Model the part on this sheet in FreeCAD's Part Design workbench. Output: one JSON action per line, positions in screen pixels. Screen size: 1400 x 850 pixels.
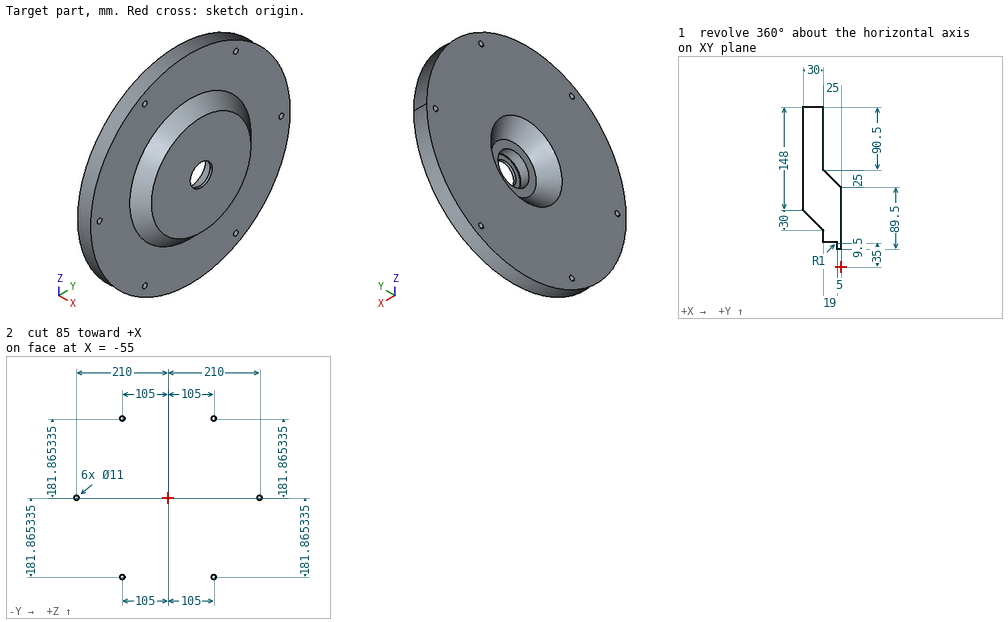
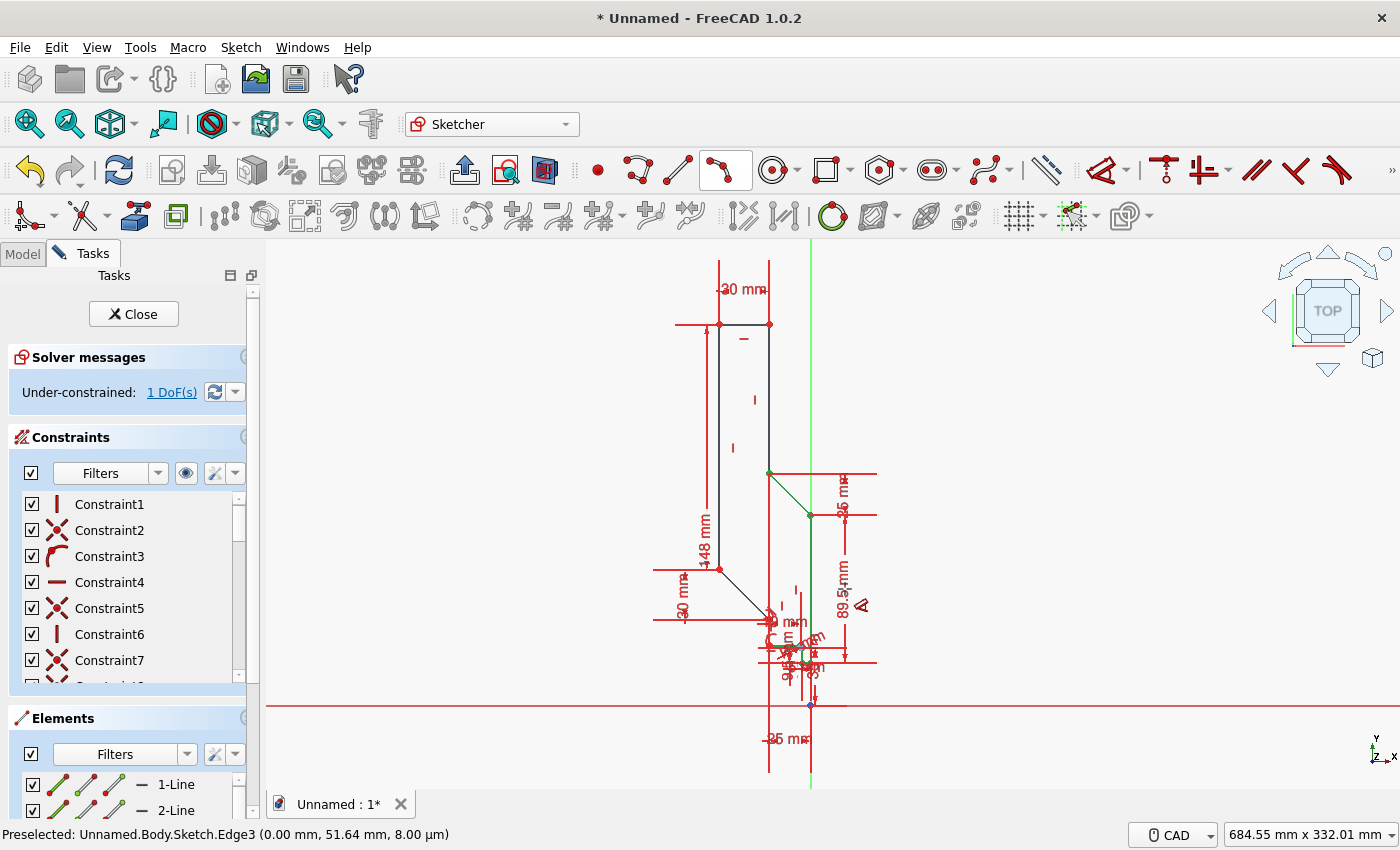
{"action": "left_click", "coordinate": [769, 429]}
{"action": "left_click", "coordinate": [735, 399]}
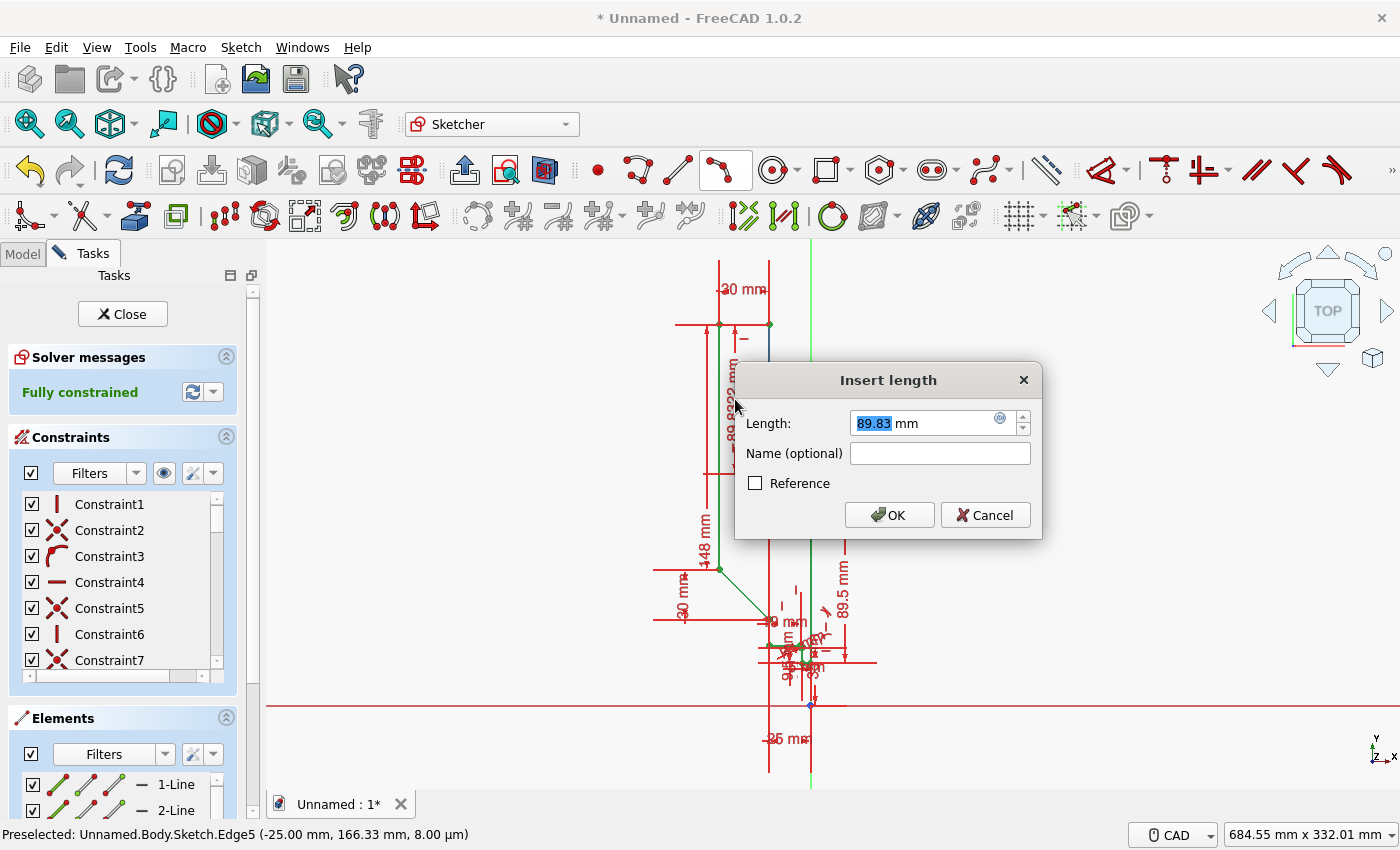
{"action": "type", "text": "90.5"}
{"action": "key", "text": "Return"}
{"action": "key", "text": "Escape"}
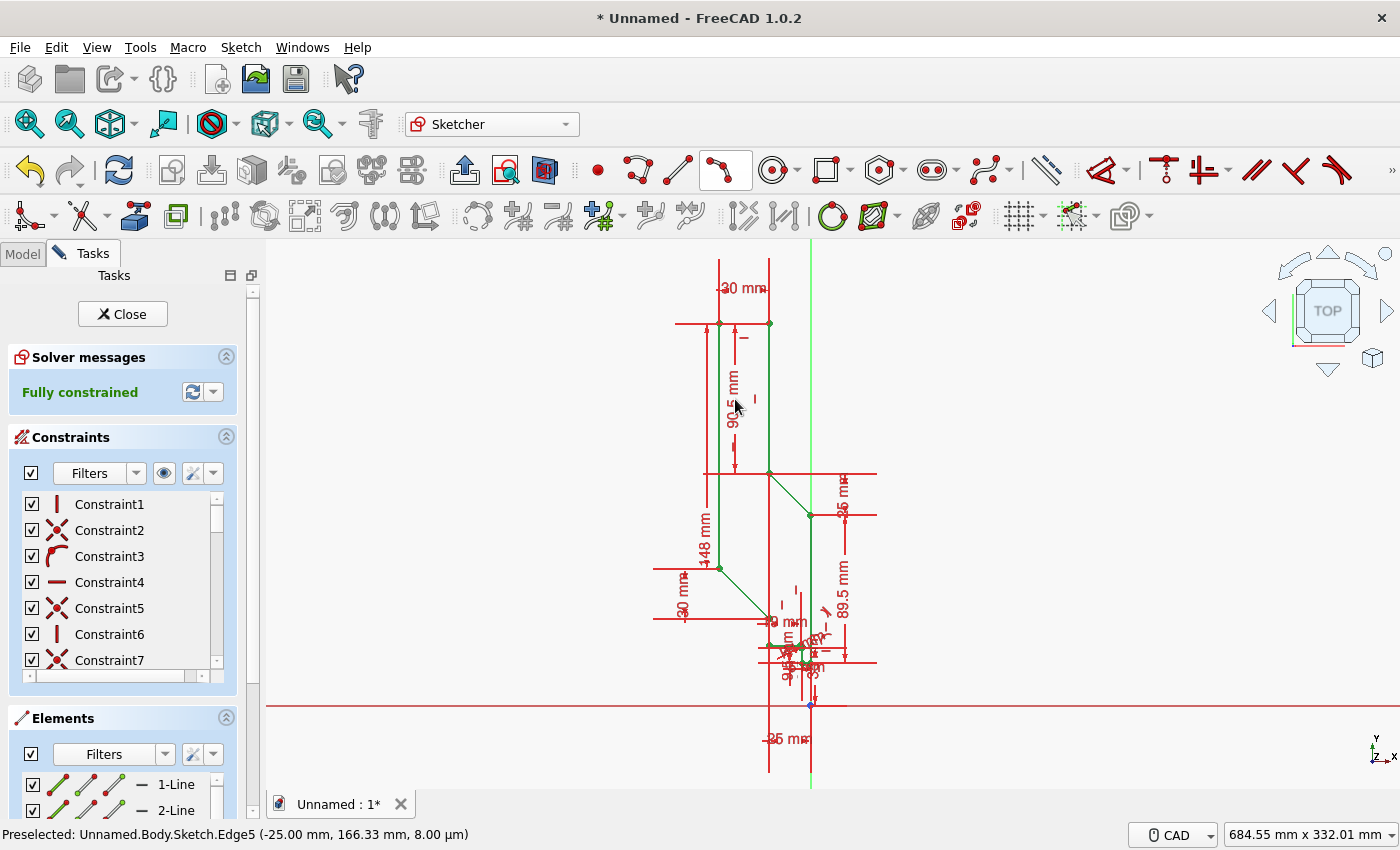
{"action": "left_click", "coordinate": [123, 314]}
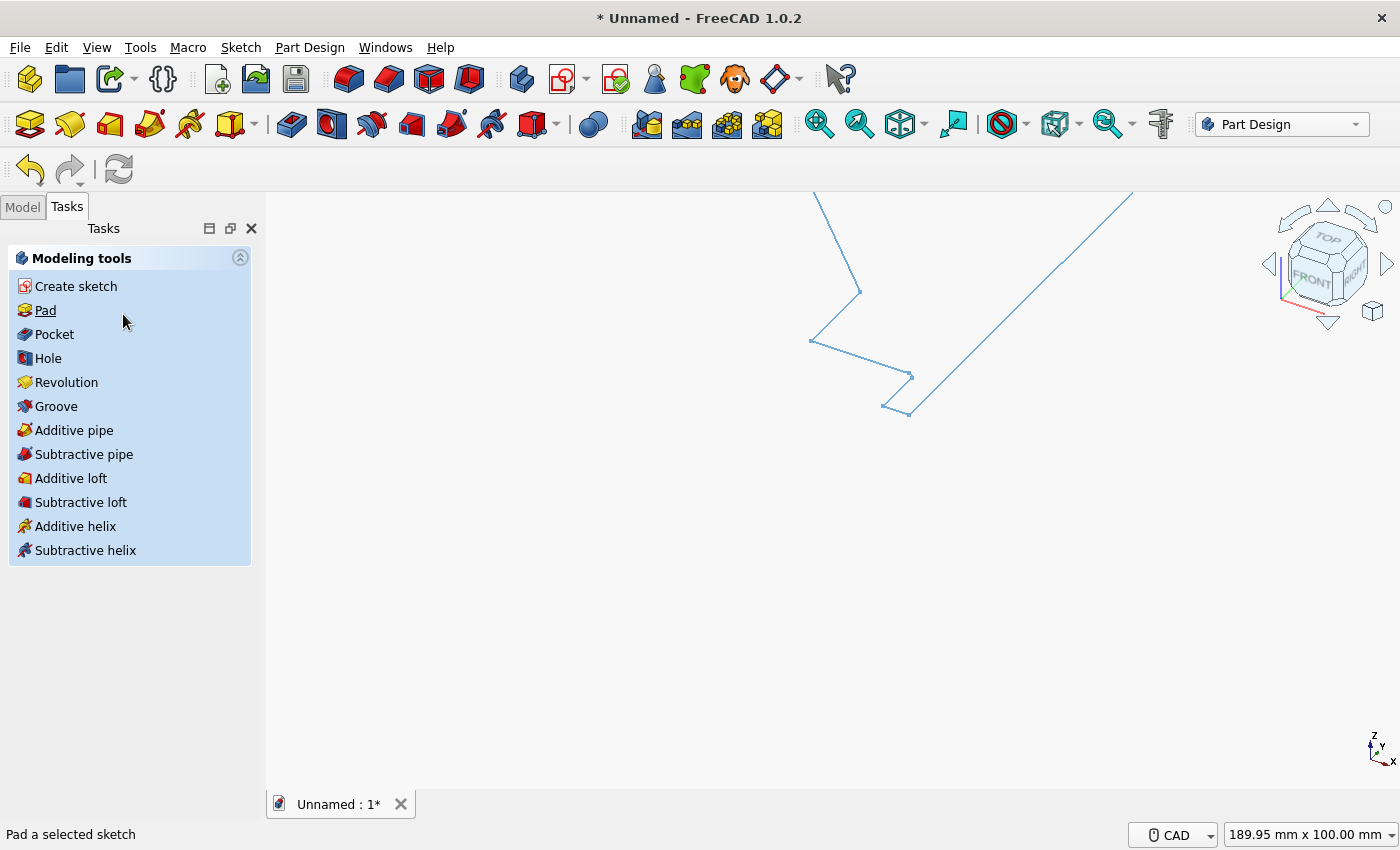
{"action": "left_click", "coordinate": [70, 124]}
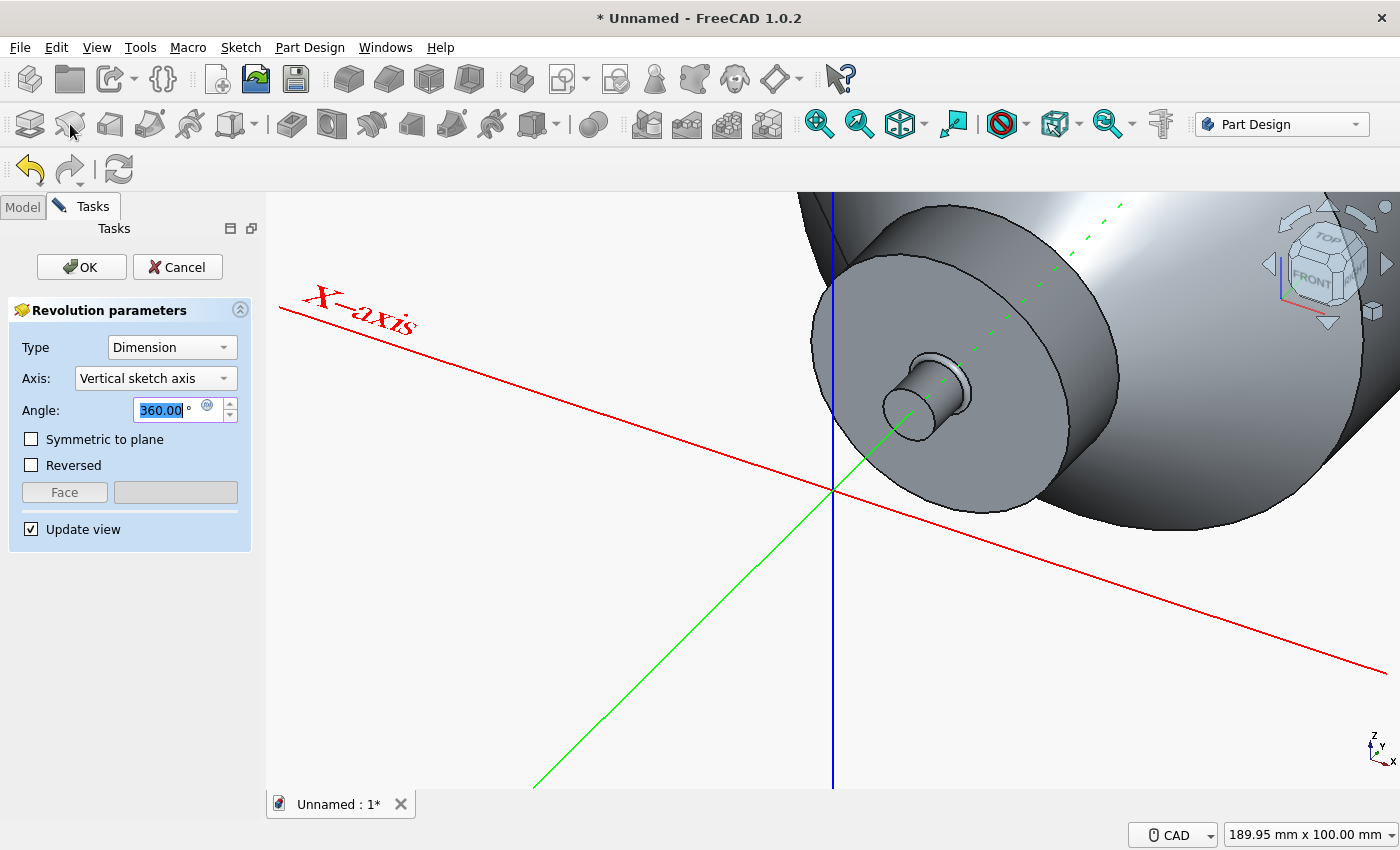
{"action": "left_click", "coordinate": [156, 378]}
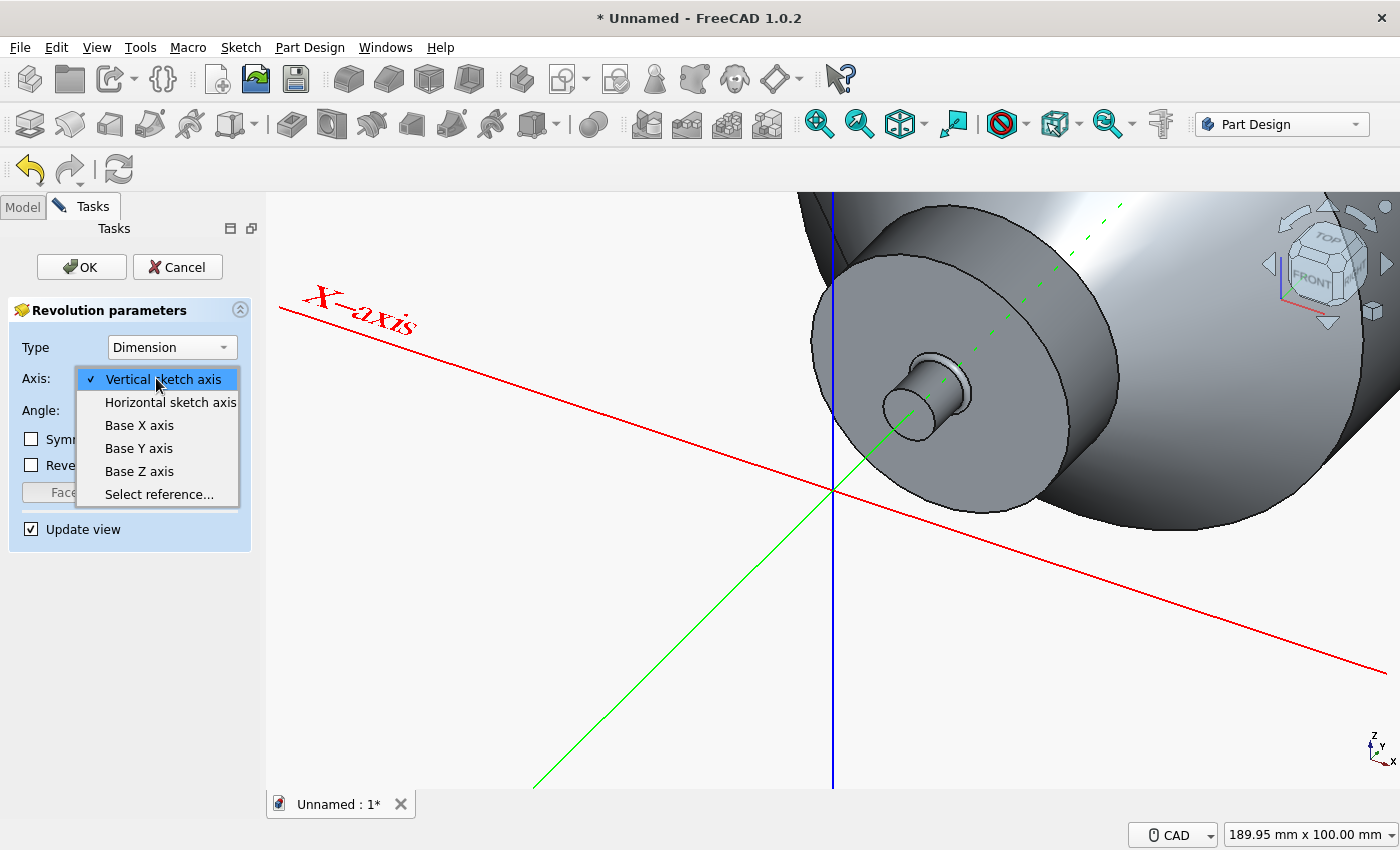
{"action": "left_click", "coordinate": [156, 402]}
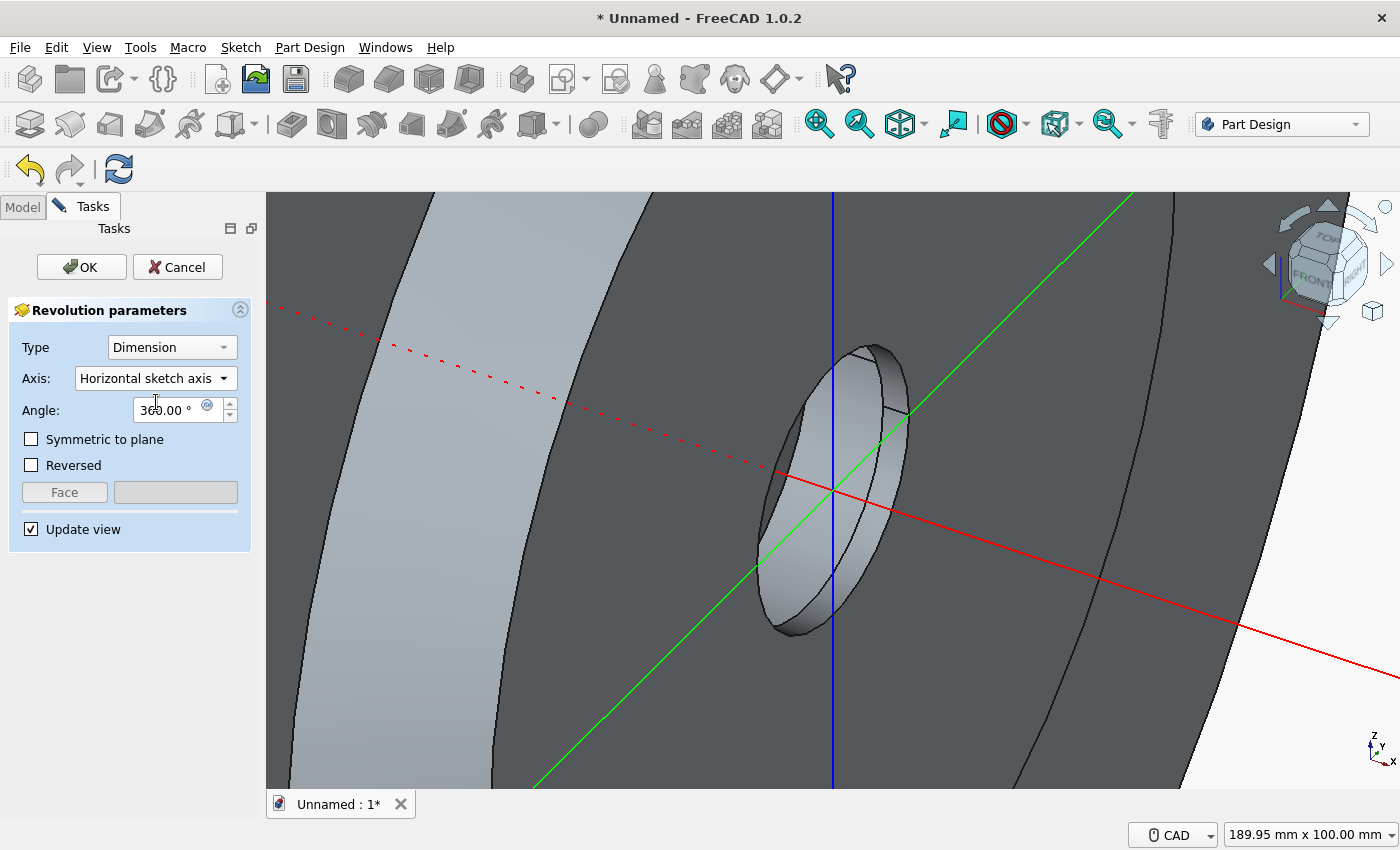
{"action": "left_click", "coordinate": [82, 267]}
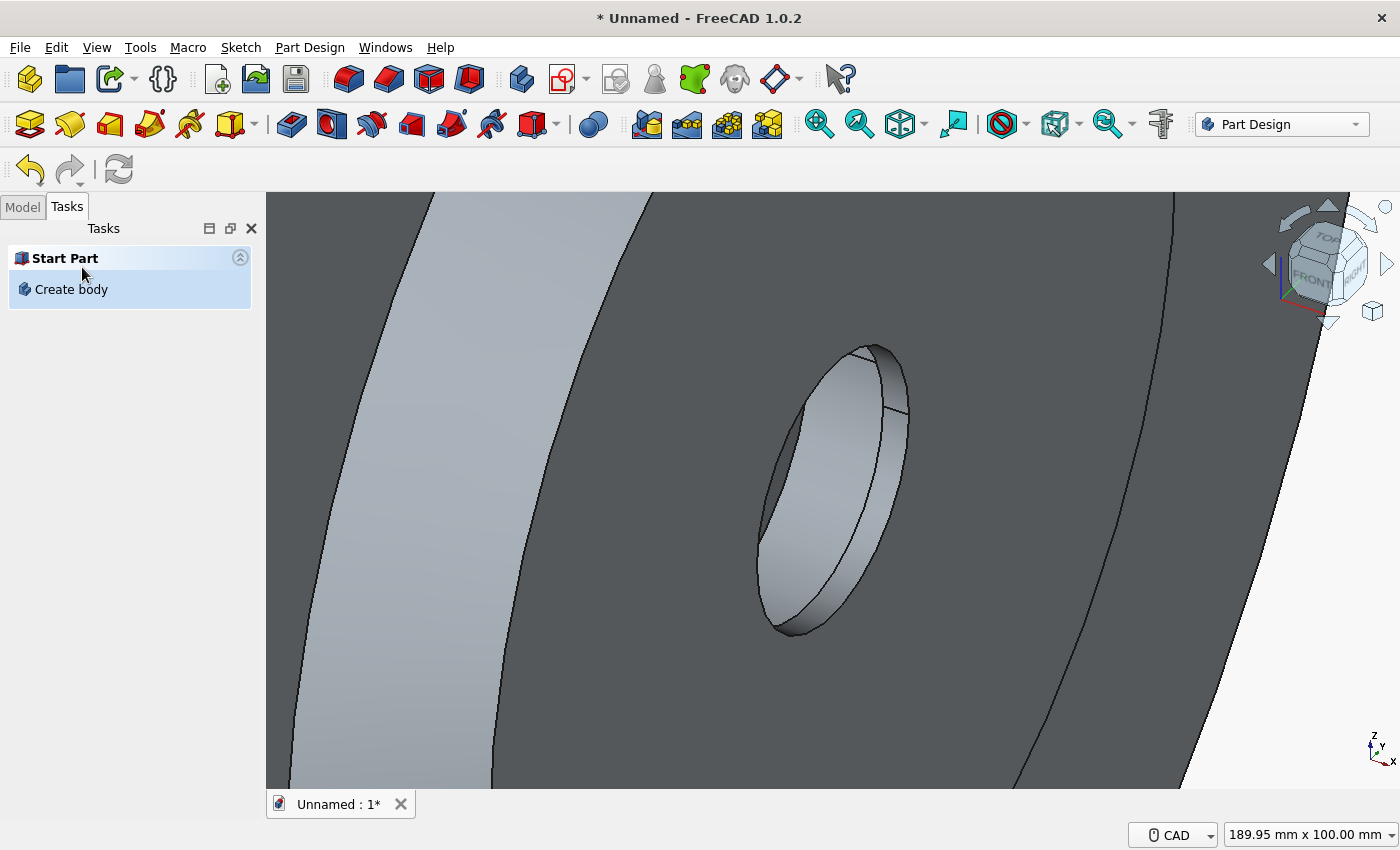
{"action": "left_click", "coordinate": [820, 124]}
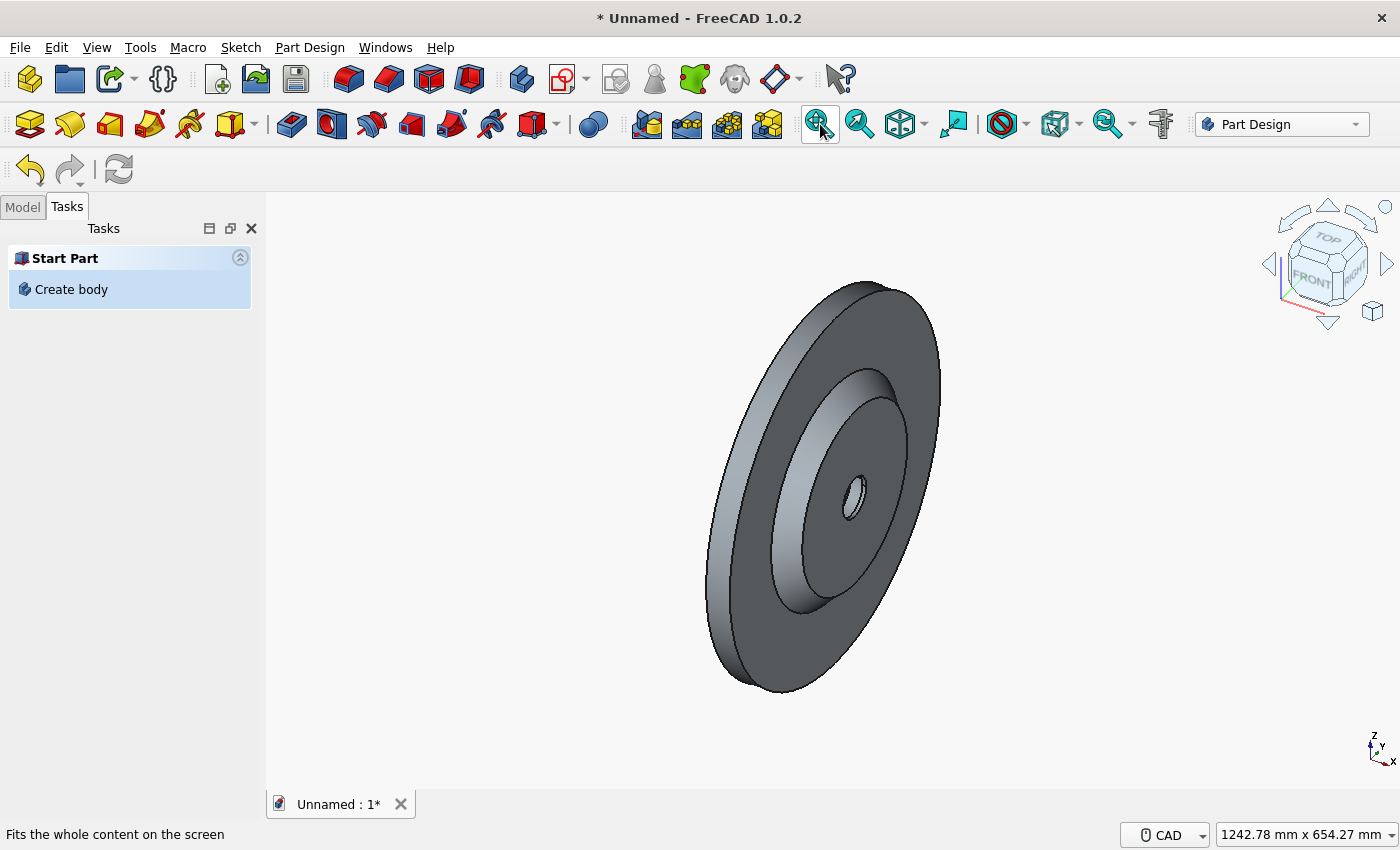
{"action": "key", "text": "6"}